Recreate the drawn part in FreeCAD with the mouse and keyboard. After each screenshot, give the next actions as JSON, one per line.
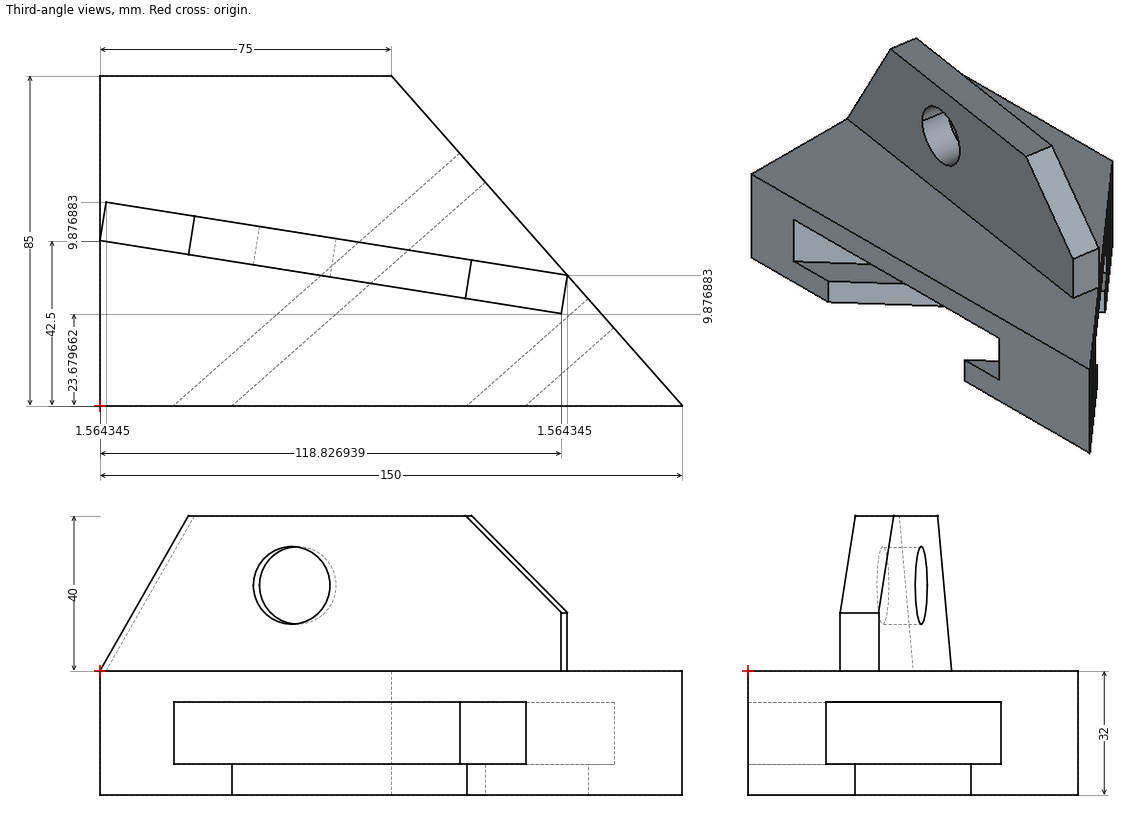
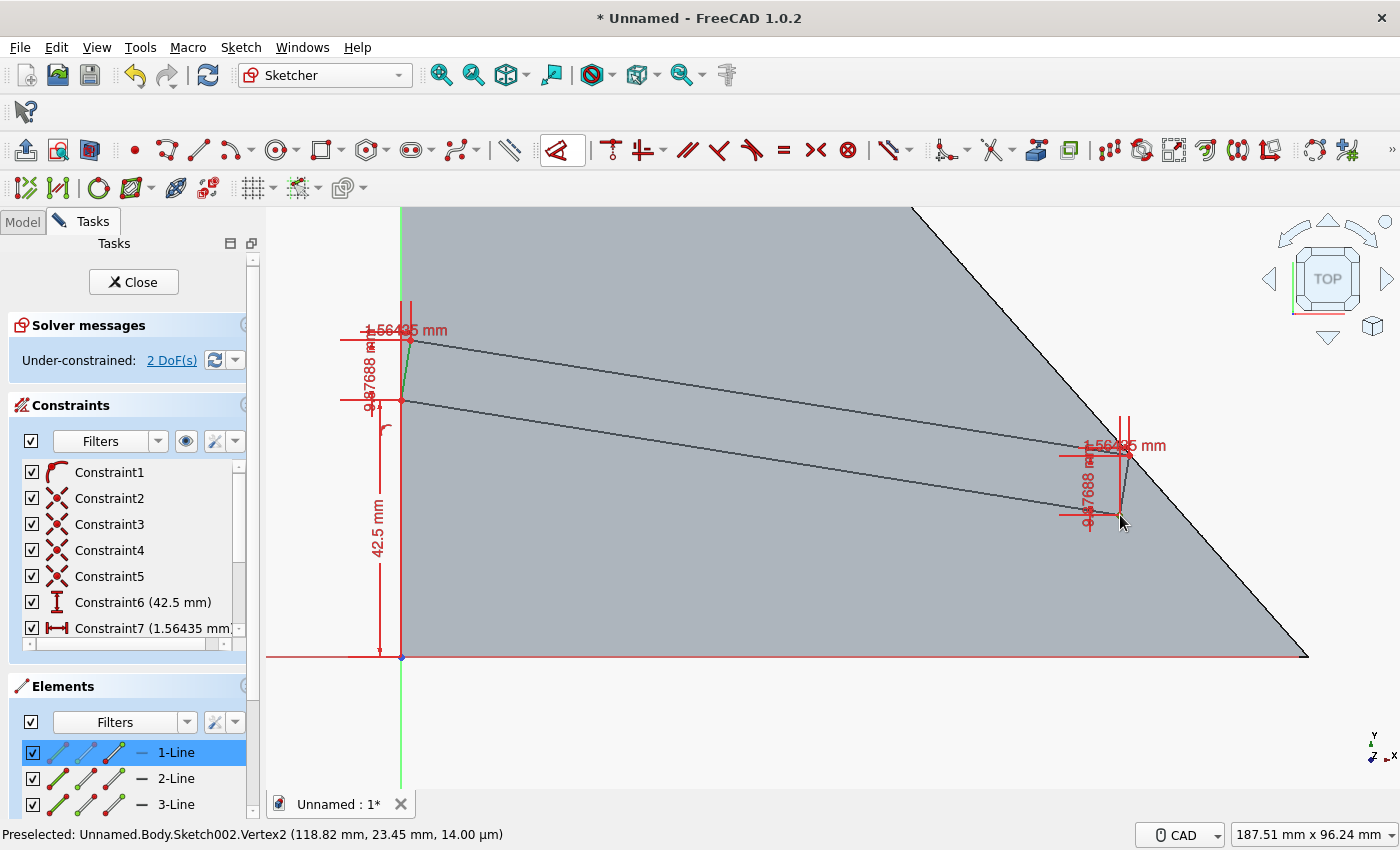
{"action": "key", "text": "i"}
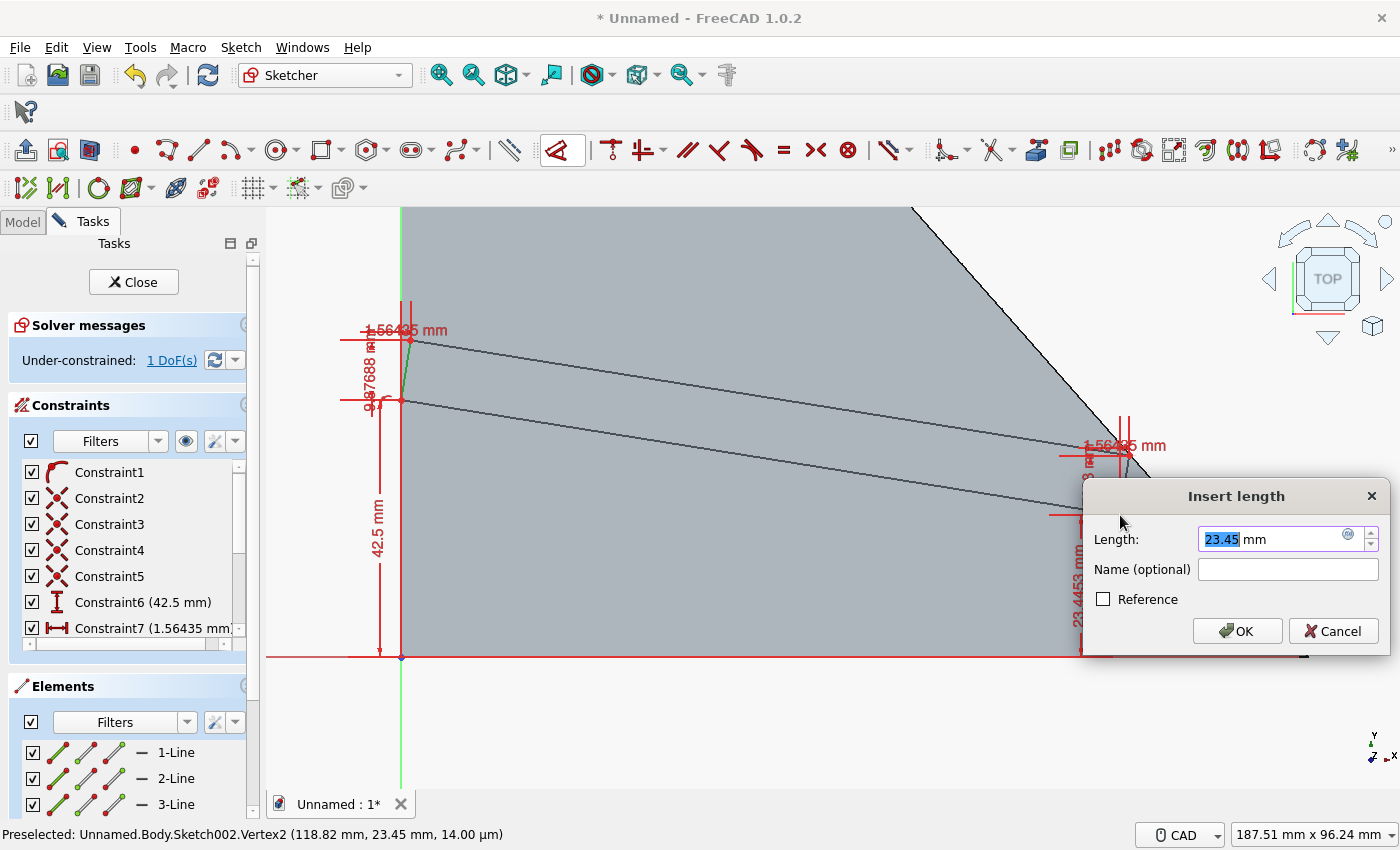
{"action": "type", "text": "23.679662"}
{"action": "key", "text": "Return"}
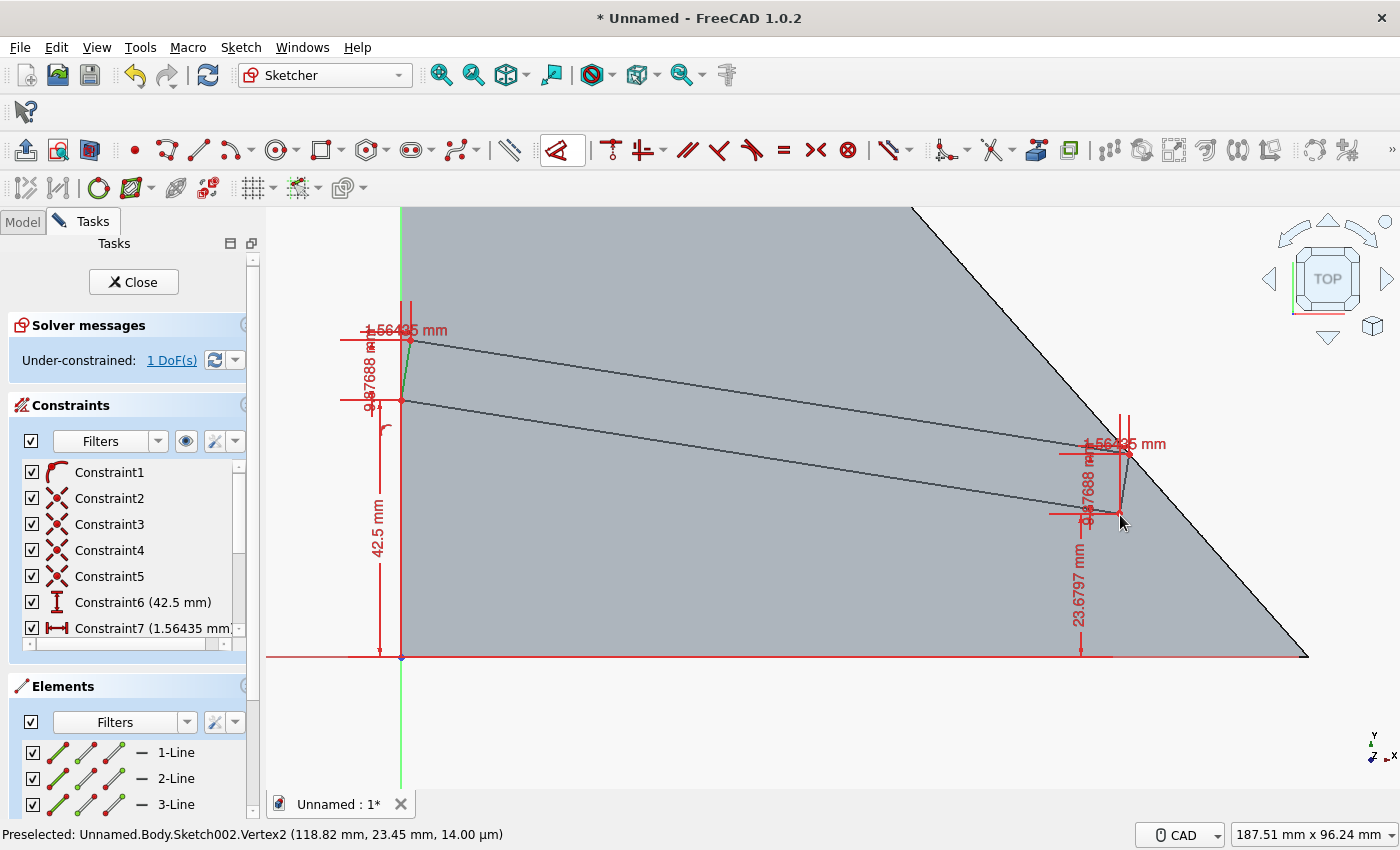
{"action": "left_click", "coordinate": [1120, 514]}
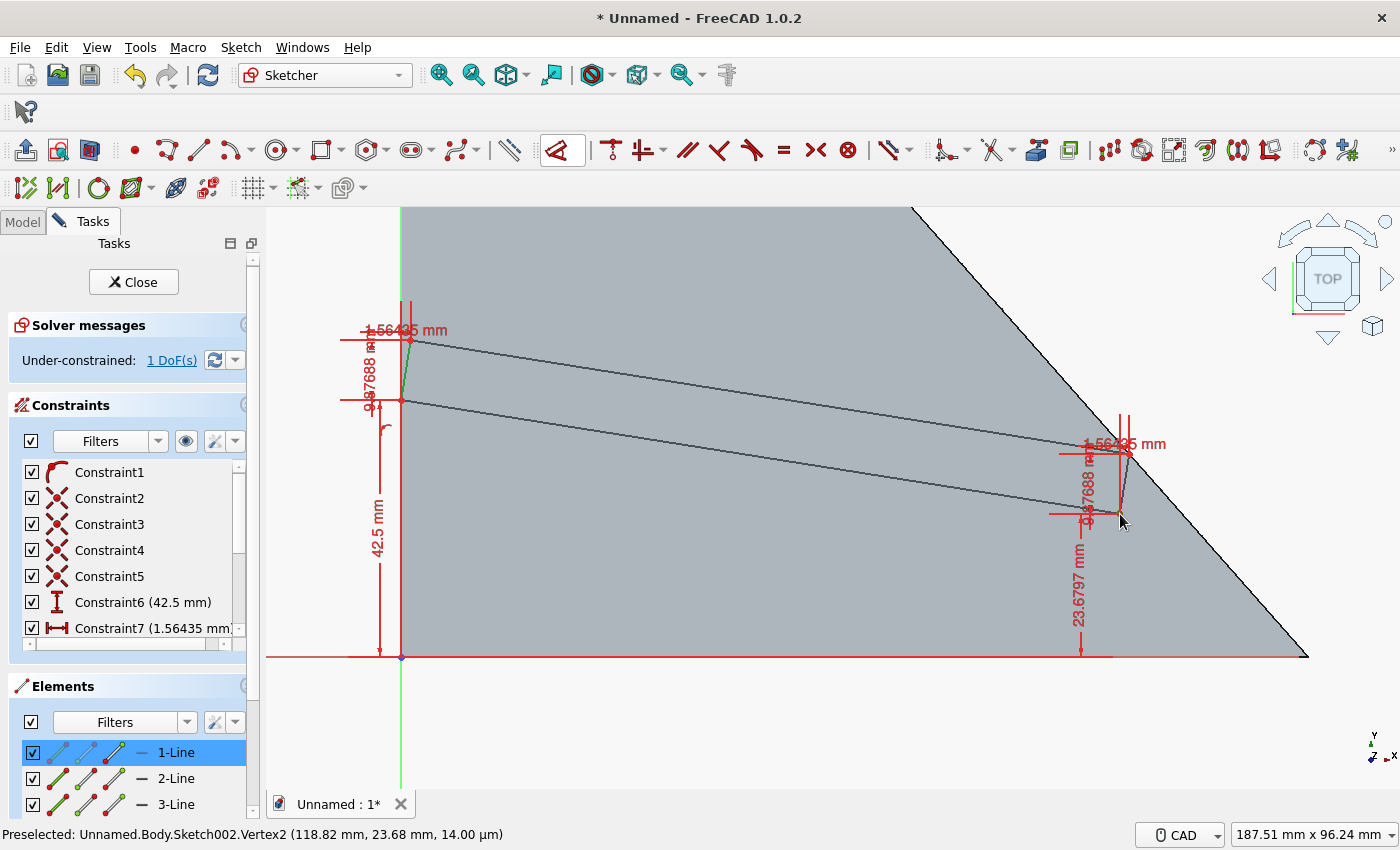
{"action": "key", "text": "l"}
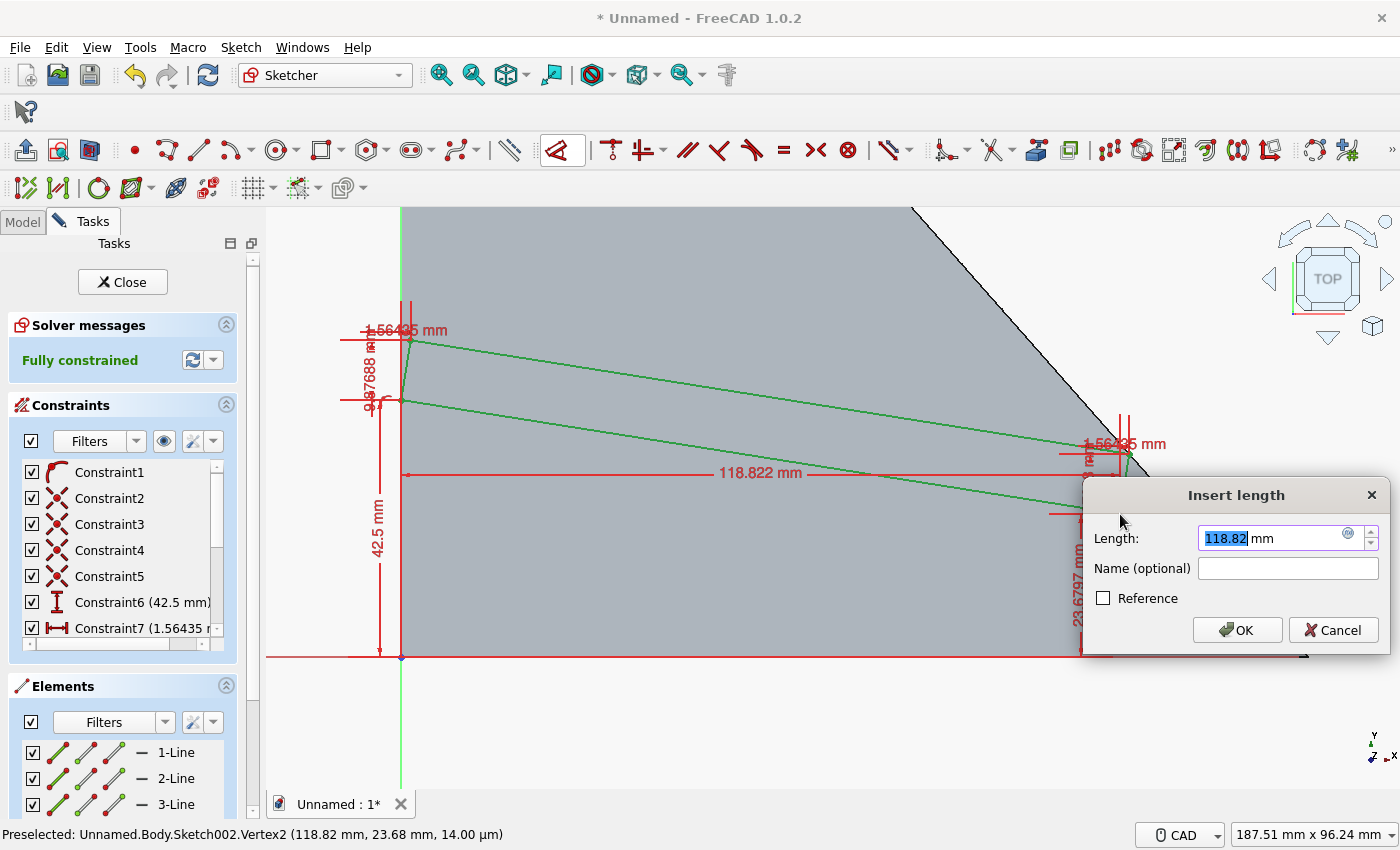
{"action": "type", "text": "118.826939"}
{"action": "key", "text": "Return"}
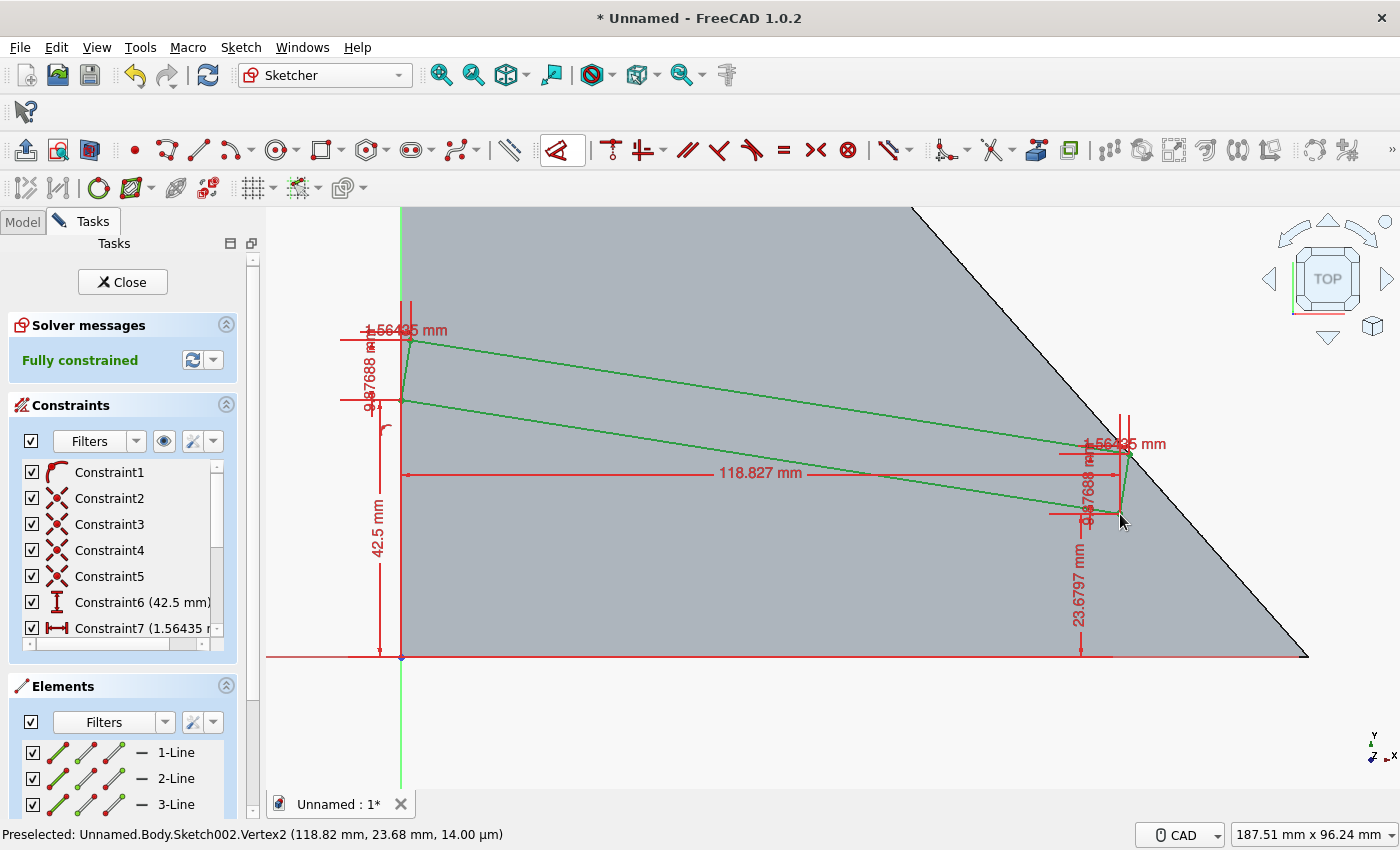
{"action": "left_click", "coordinate": [123, 282]}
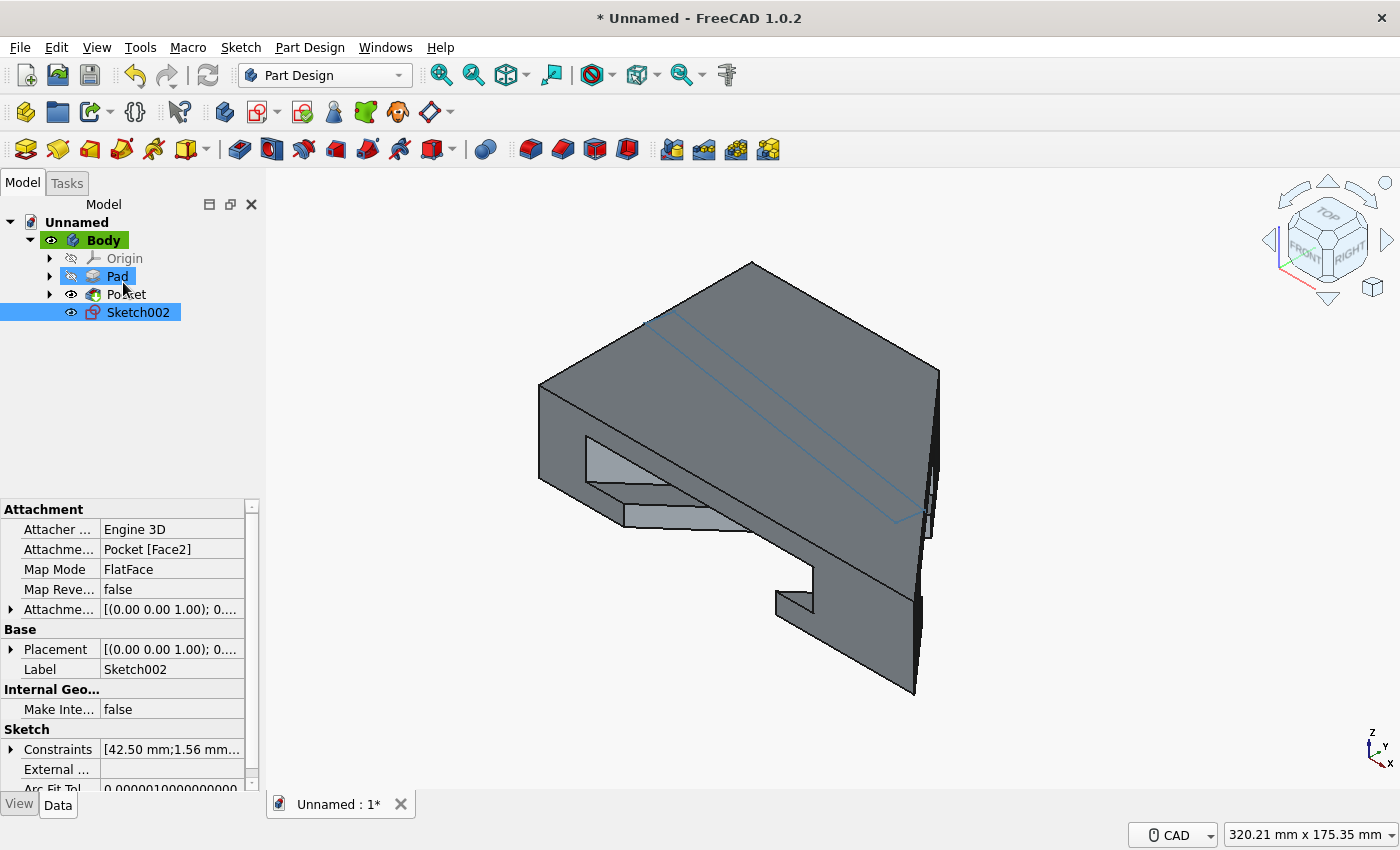
{"action": "left_click", "coordinate": [26, 150]}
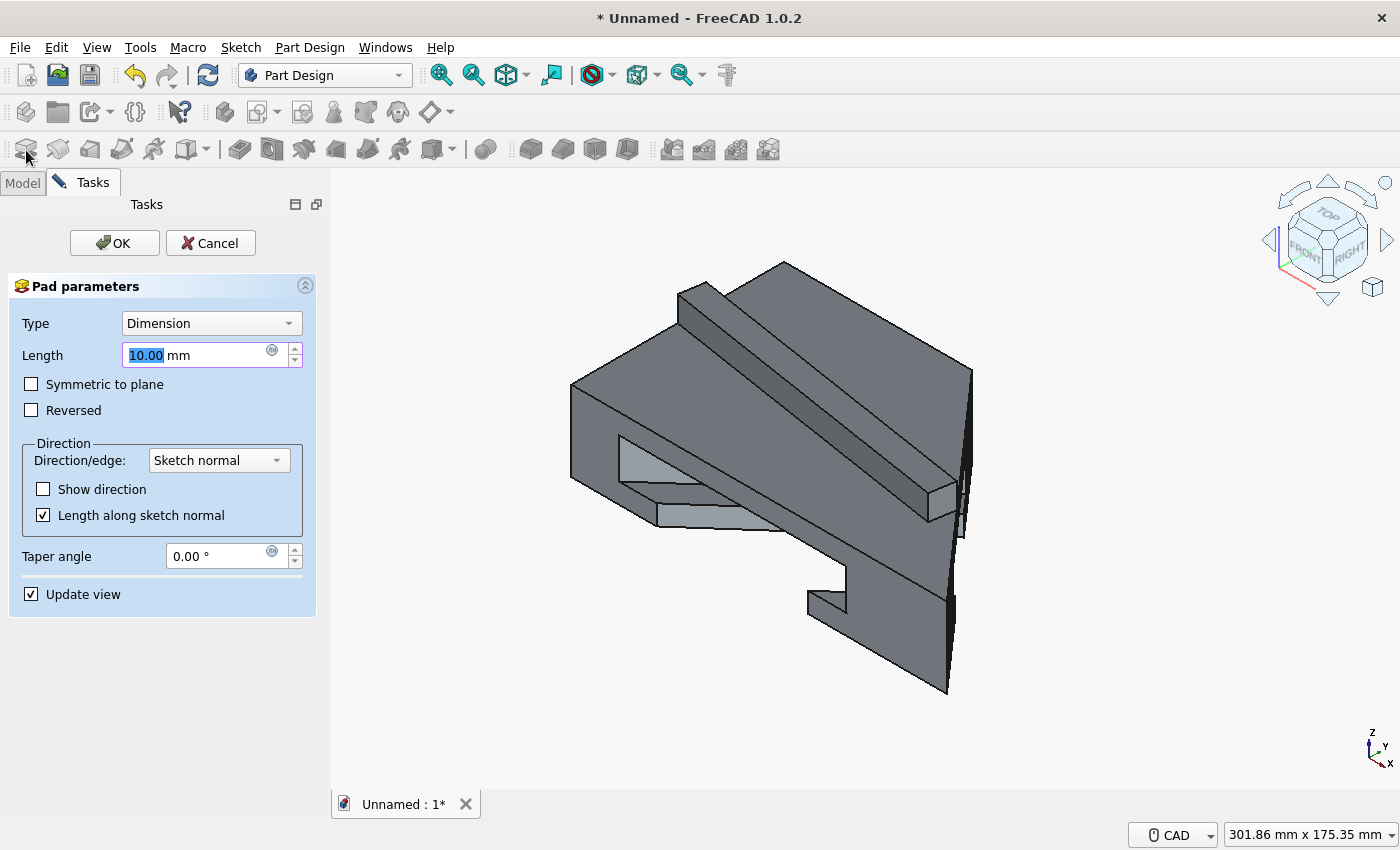
{"action": "type", "text": "40"}
{"action": "key", "text": "Tab"}